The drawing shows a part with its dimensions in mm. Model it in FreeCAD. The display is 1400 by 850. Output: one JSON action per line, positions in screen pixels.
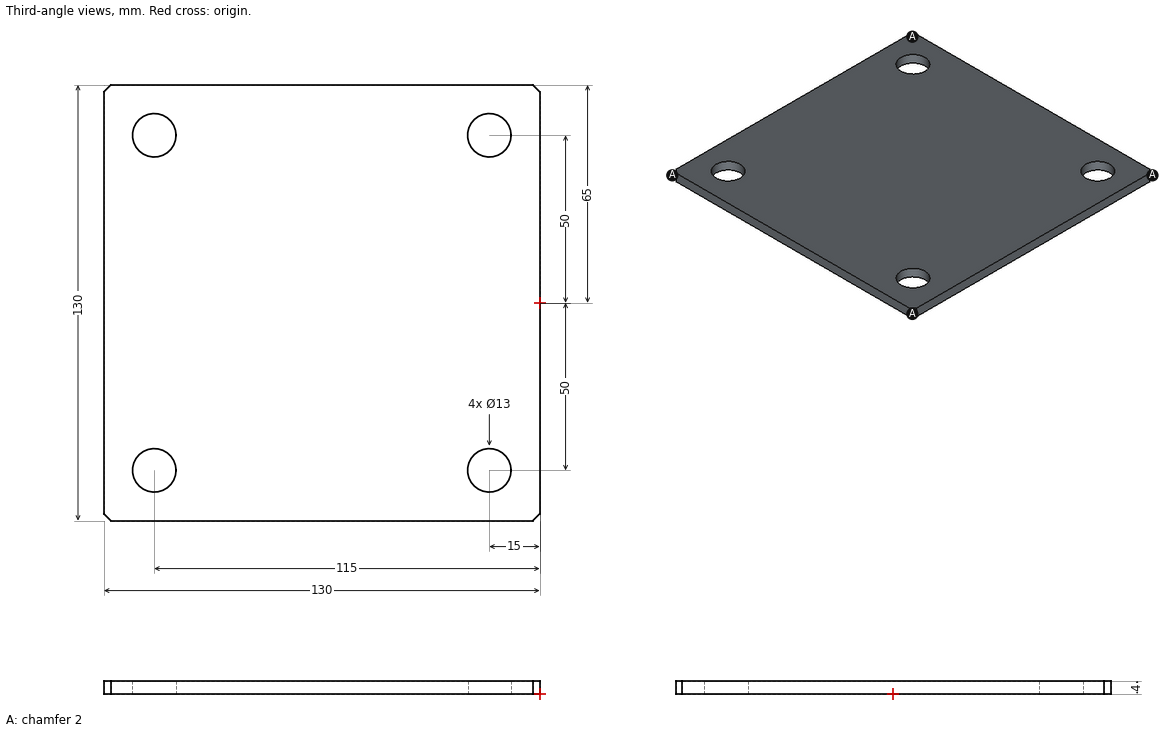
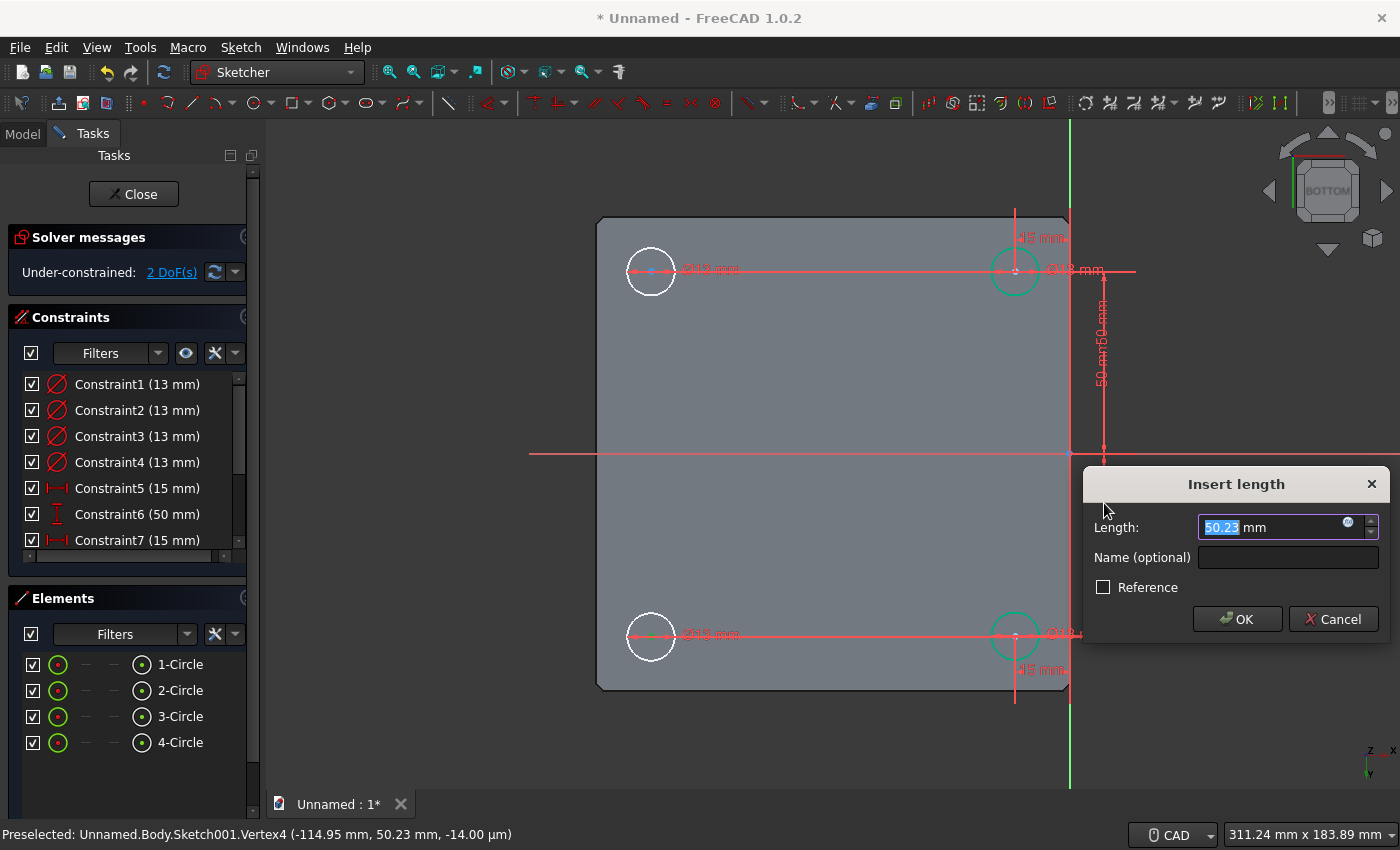
{"action": "type", "text": "50"}
{"action": "key", "text": "Return"}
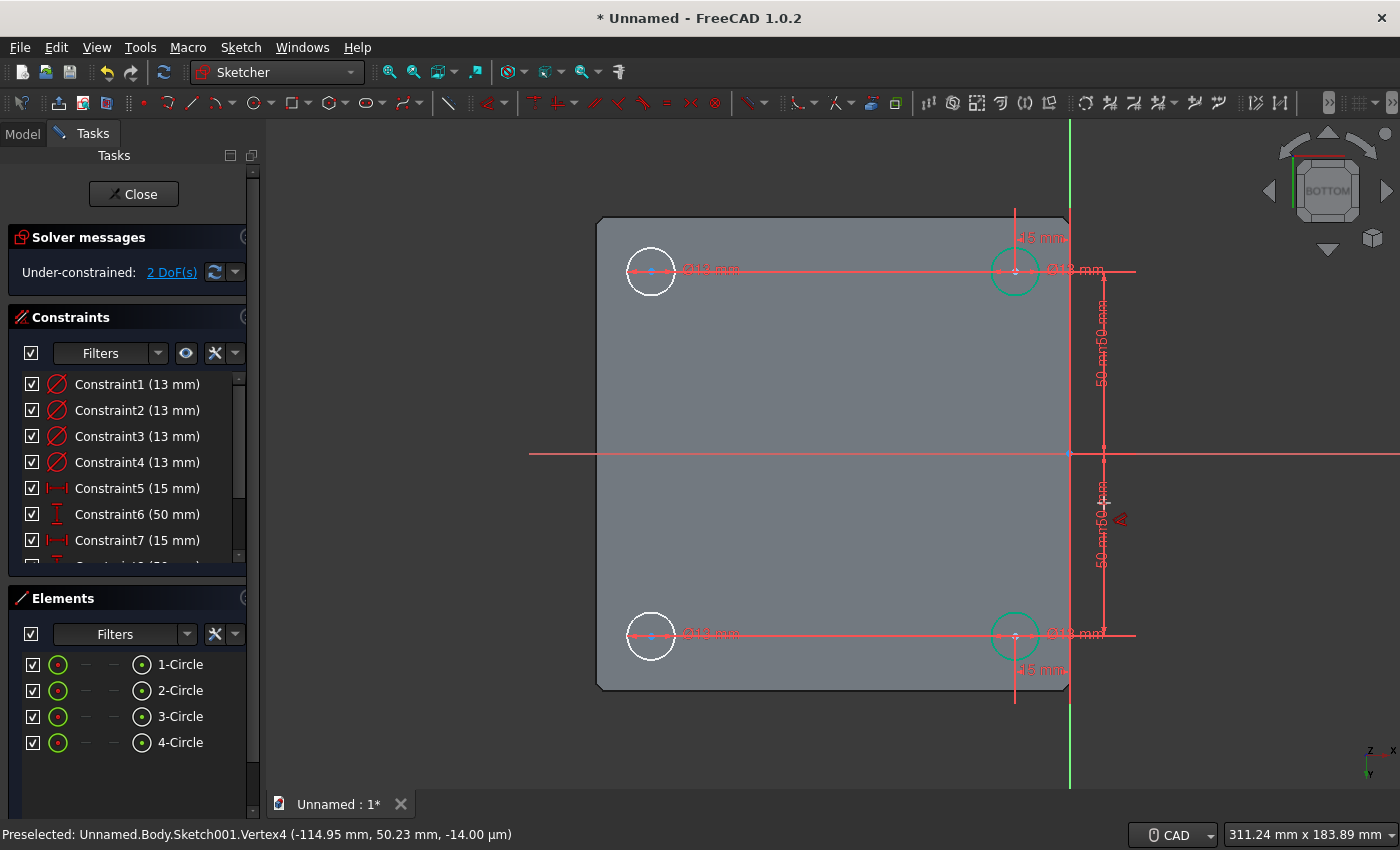
{"action": "left_click", "coordinate": [651, 272]}
{"action": "left_click", "coordinate": [860, 238]}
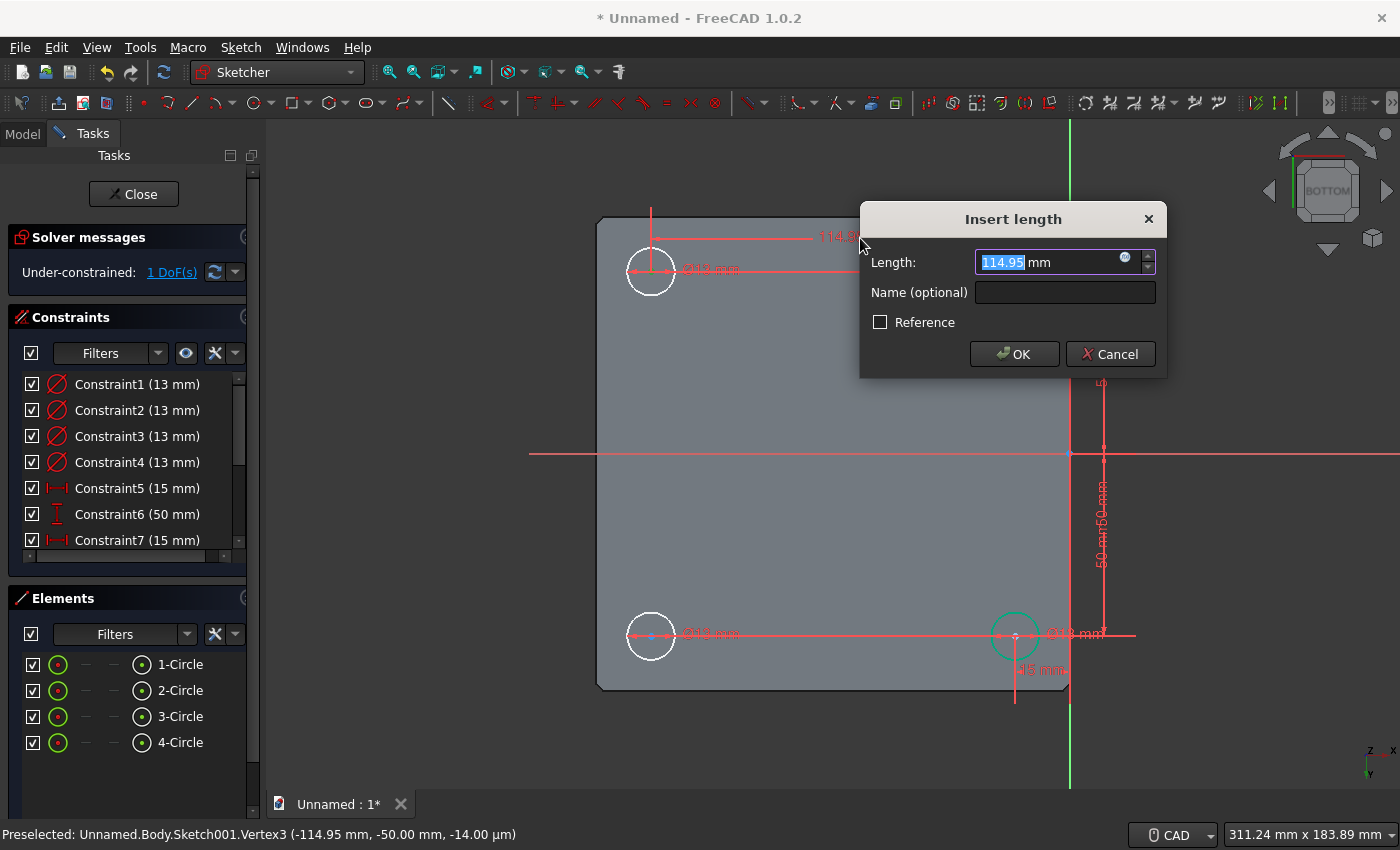
{"action": "type", "text": "115"}
{"action": "key", "text": "Return"}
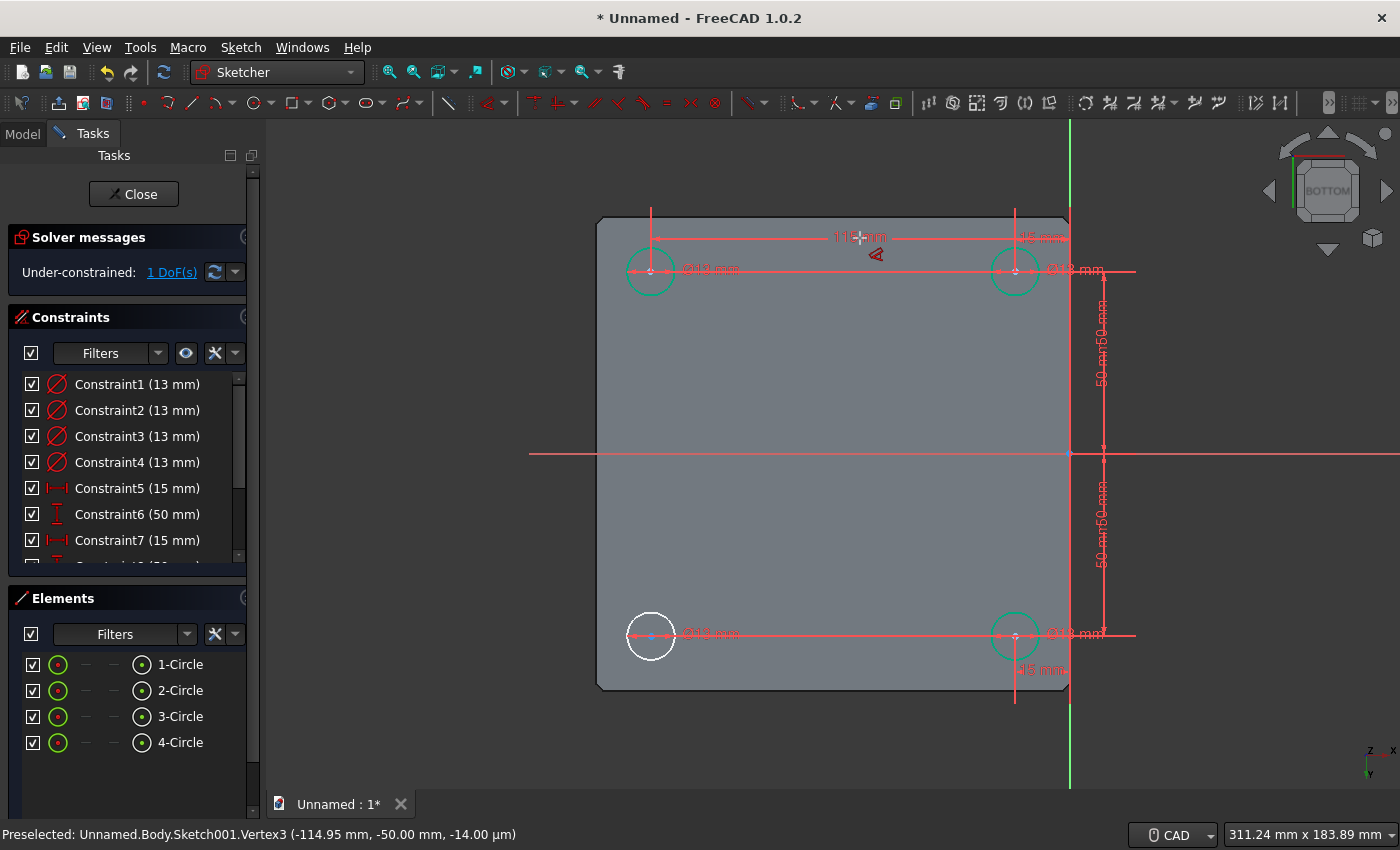
{"action": "left_click", "coordinate": [651, 636]}
{"action": "left_click", "coordinate": [860, 670]}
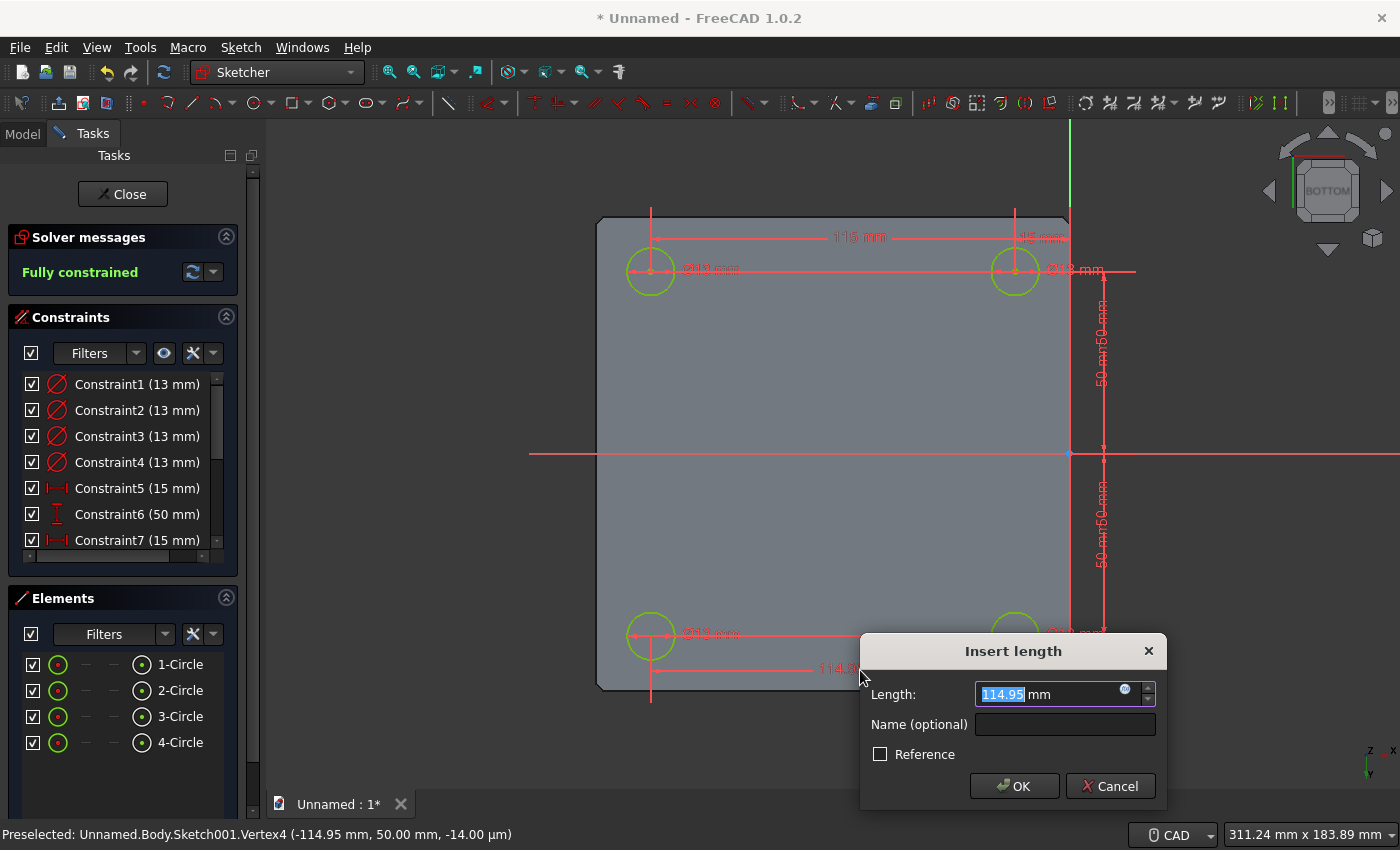
{"action": "type", "text": "115"}
{"action": "key", "text": "Return"}
{"action": "key", "text": "Escape"}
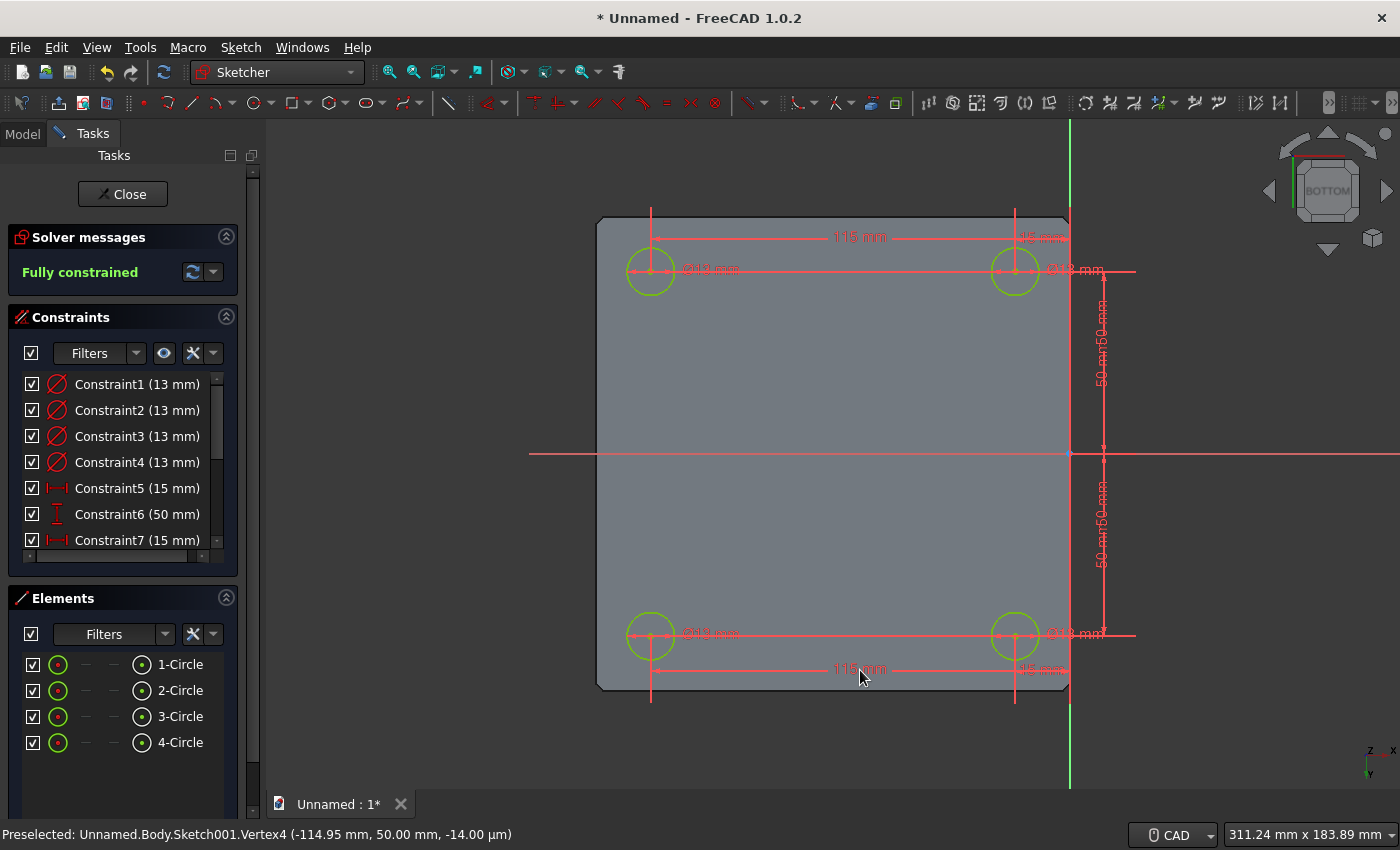
{"action": "left_click", "coordinate": [123, 194]}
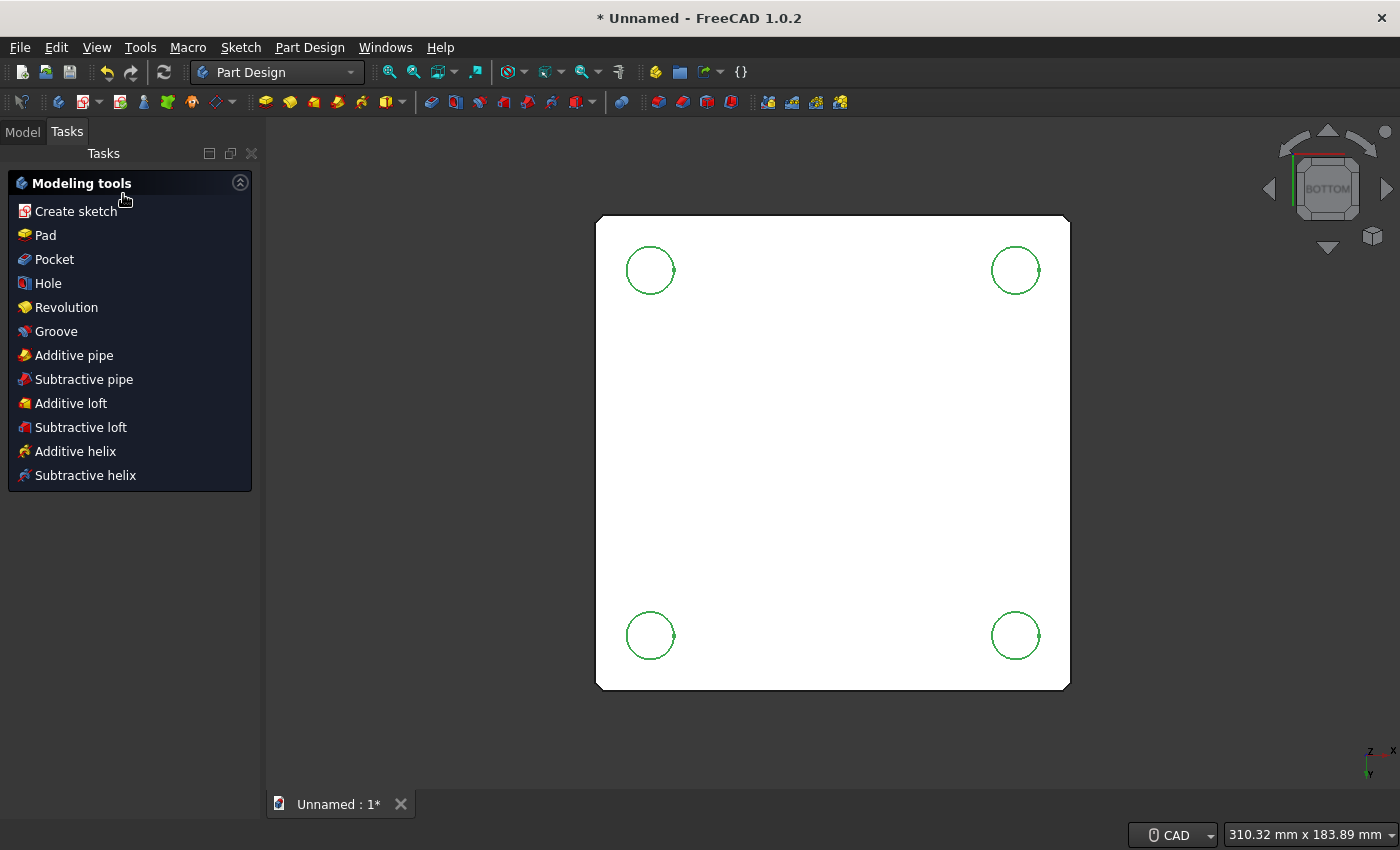
{"action": "left_click", "coordinate": [432, 102]}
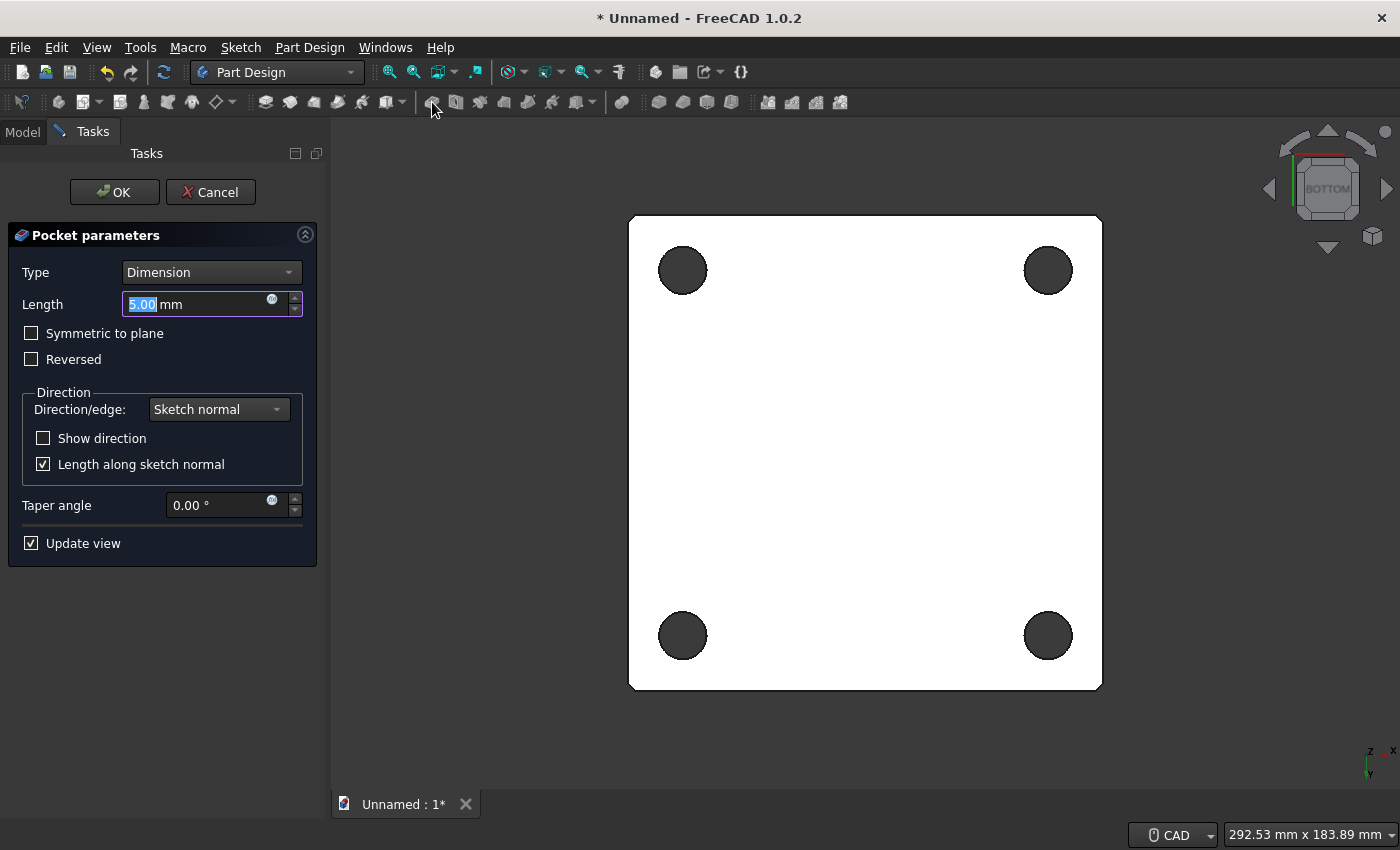
{"action": "left_click", "coordinate": [212, 272]}